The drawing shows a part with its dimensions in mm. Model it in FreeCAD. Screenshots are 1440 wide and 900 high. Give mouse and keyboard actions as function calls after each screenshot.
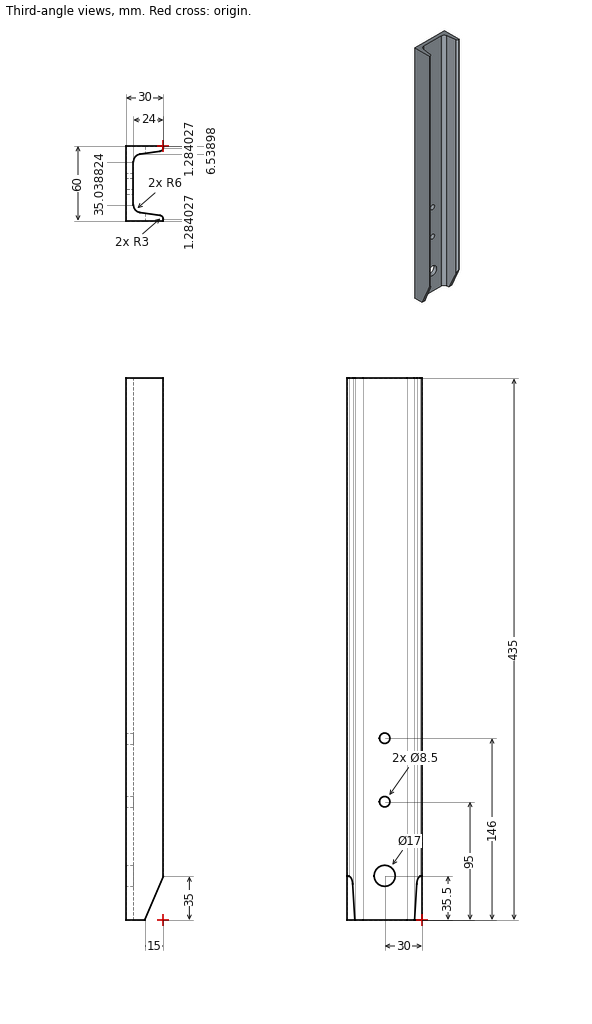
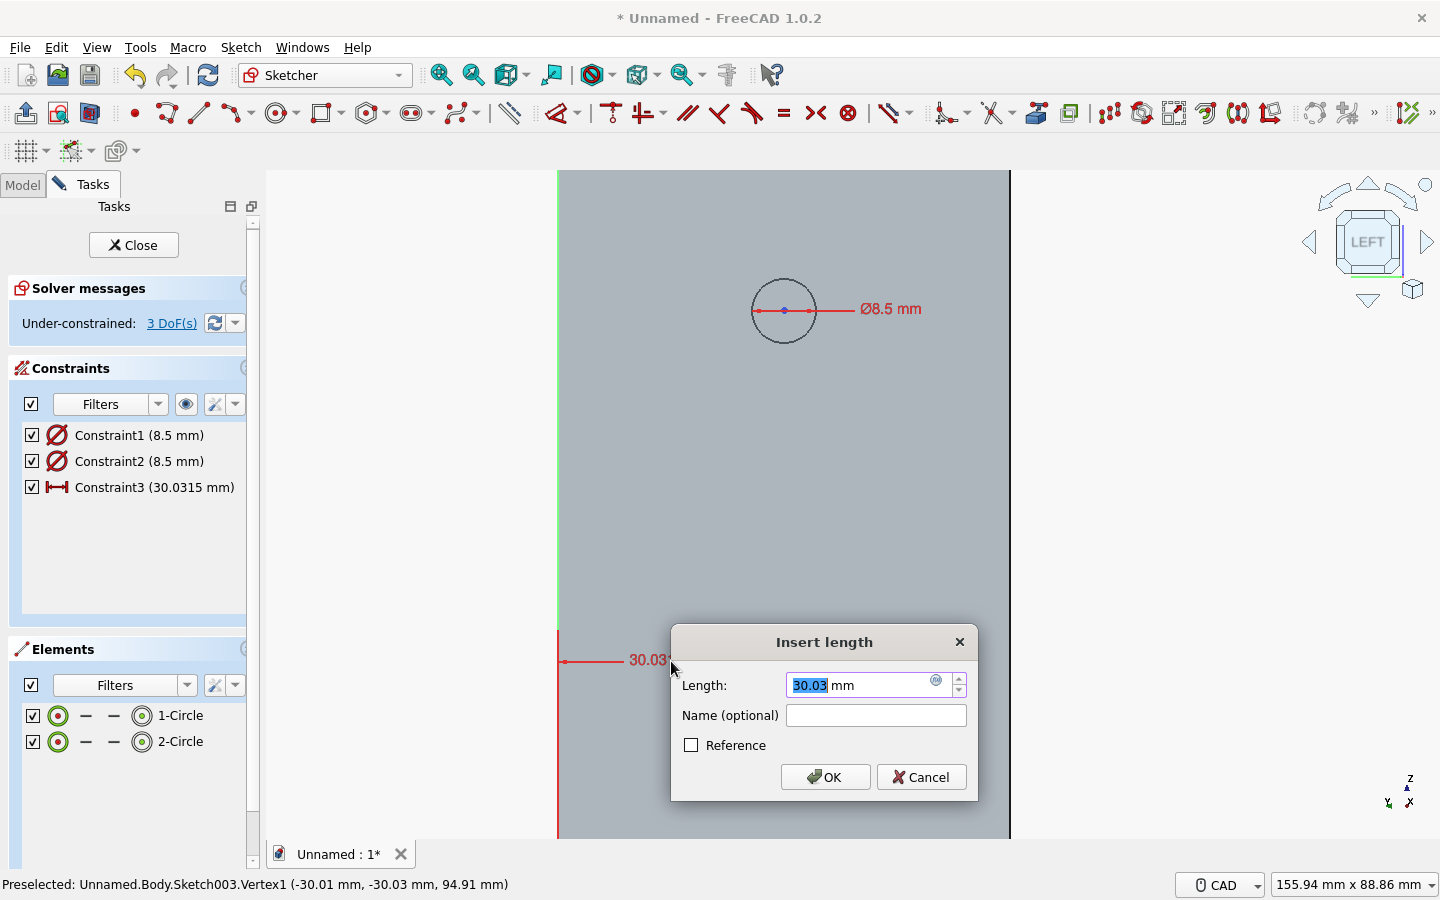
text(30)
key(Return)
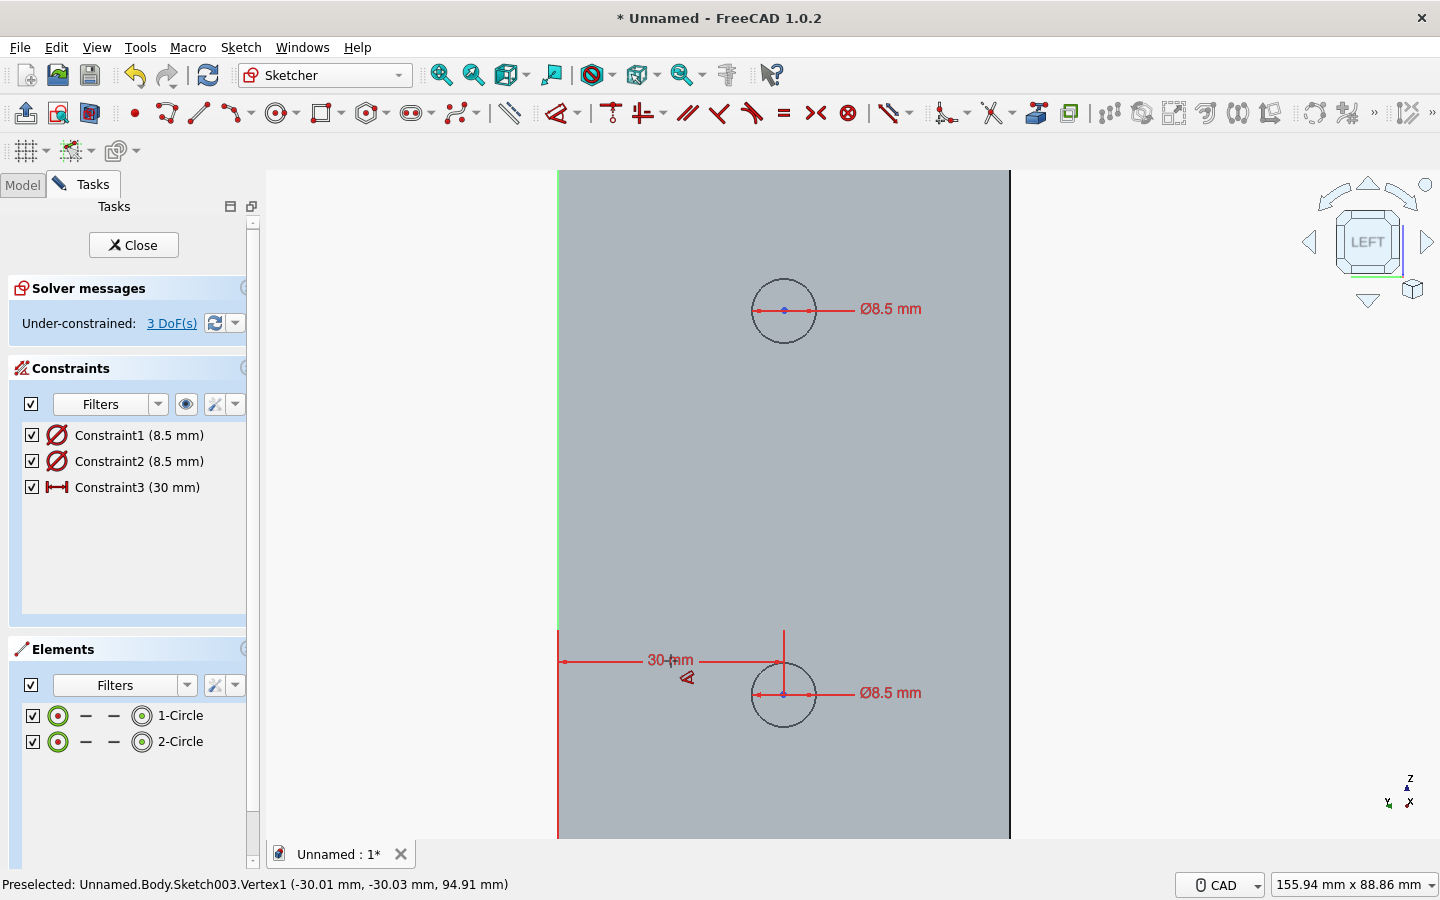
click(784, 695)
click(524, 753)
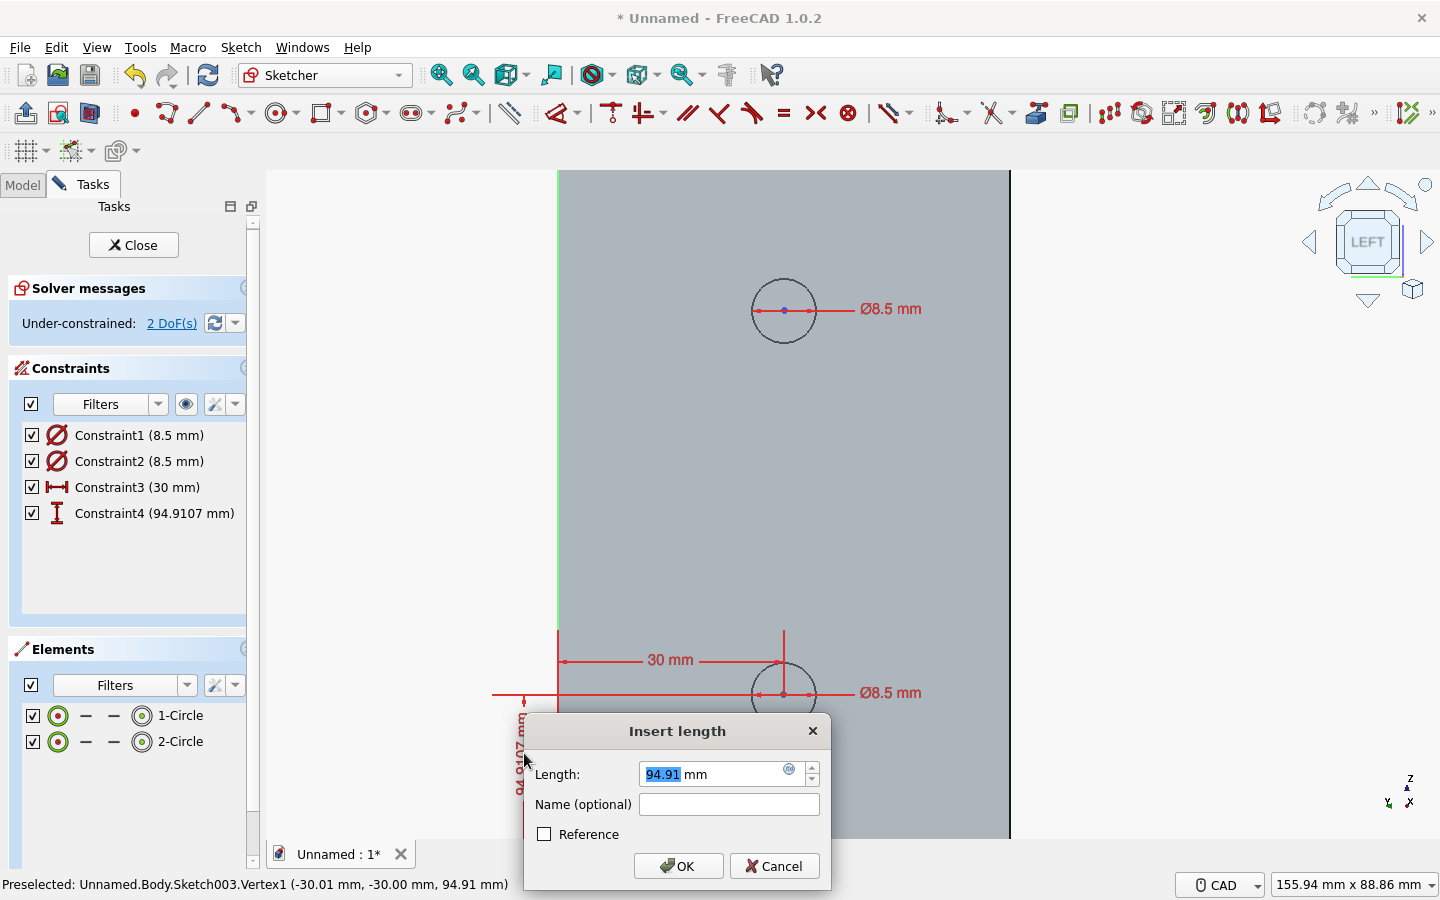
text(95)
key(Return)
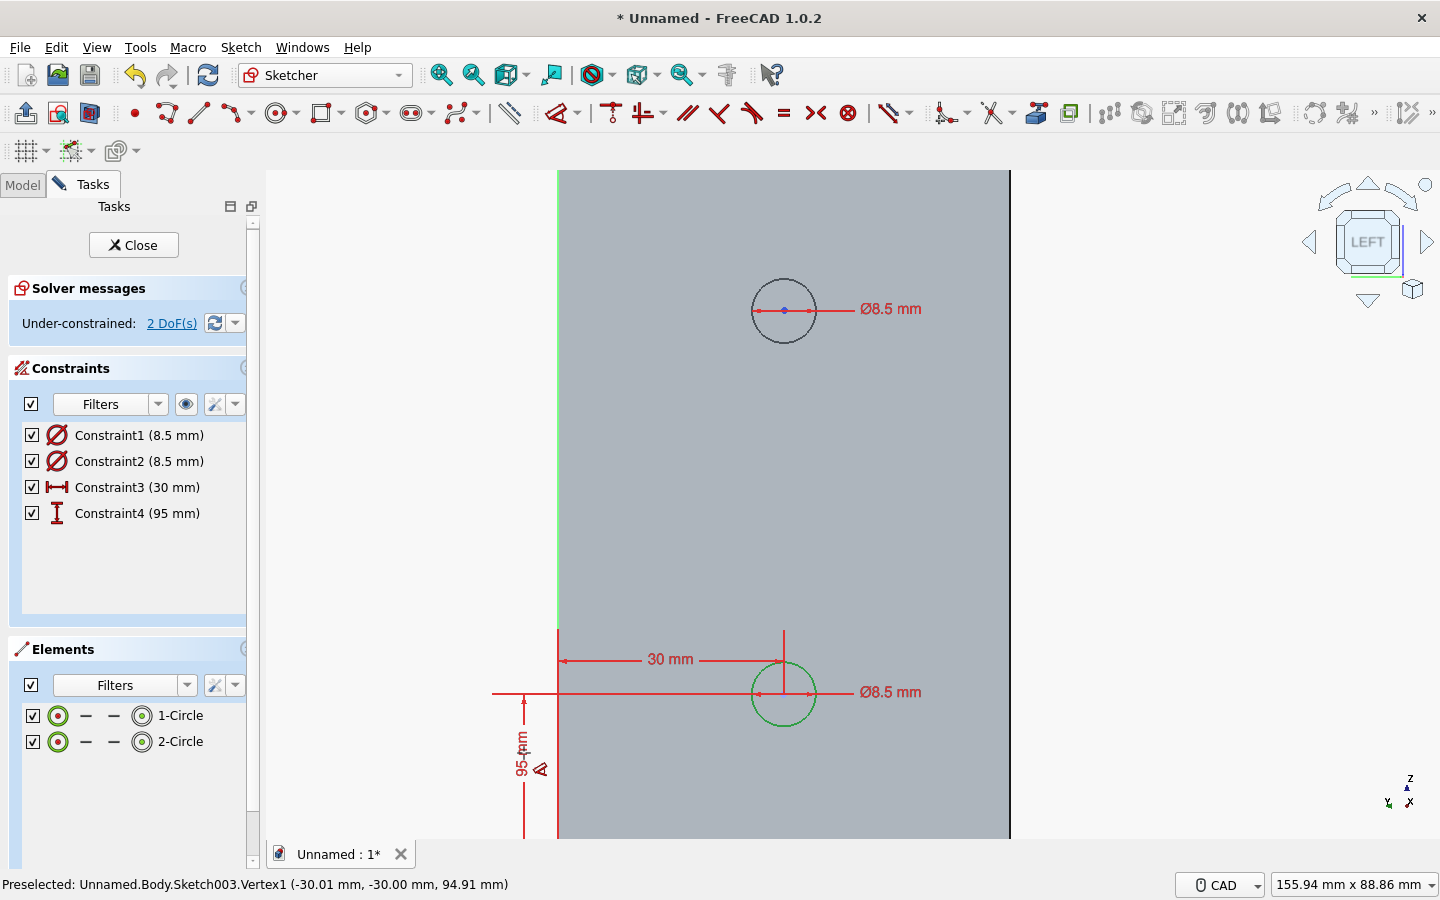
click(784, 311)
click(671, 277)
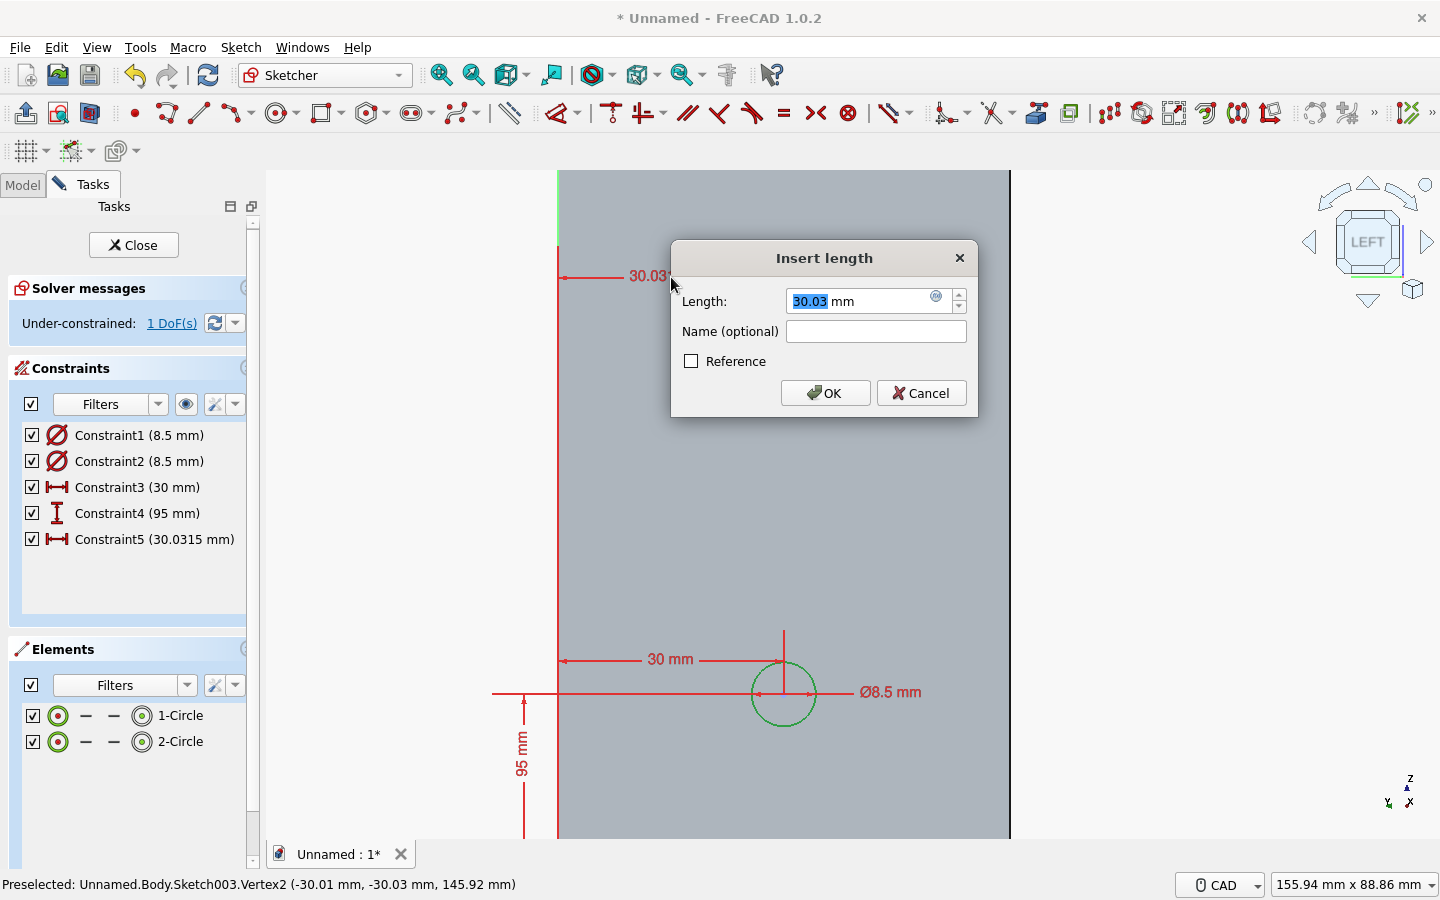
text(30)
key(Return)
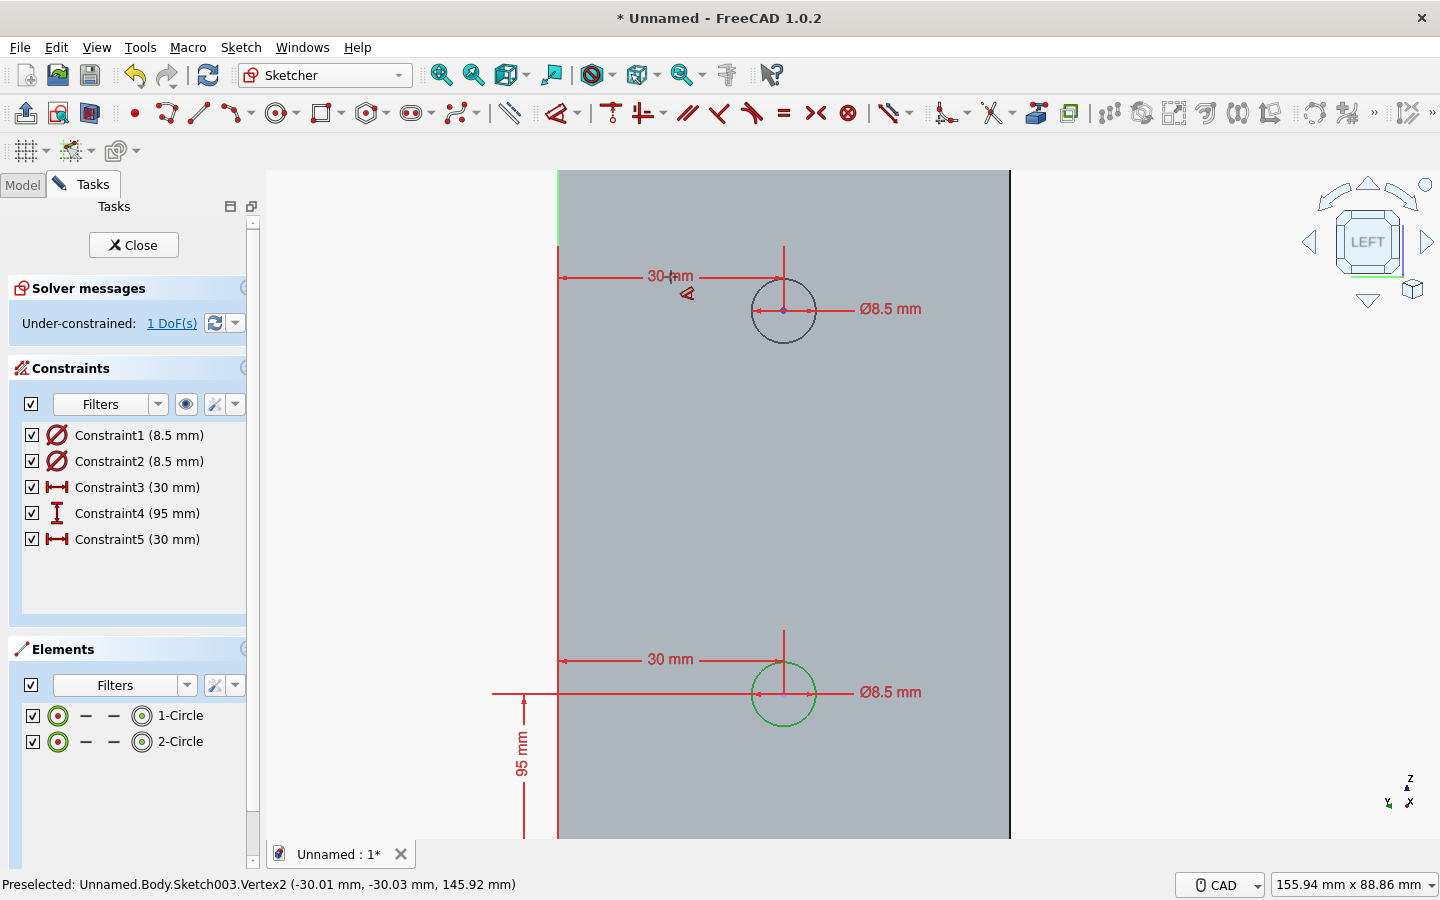
click(784, 311)
click(524, 561)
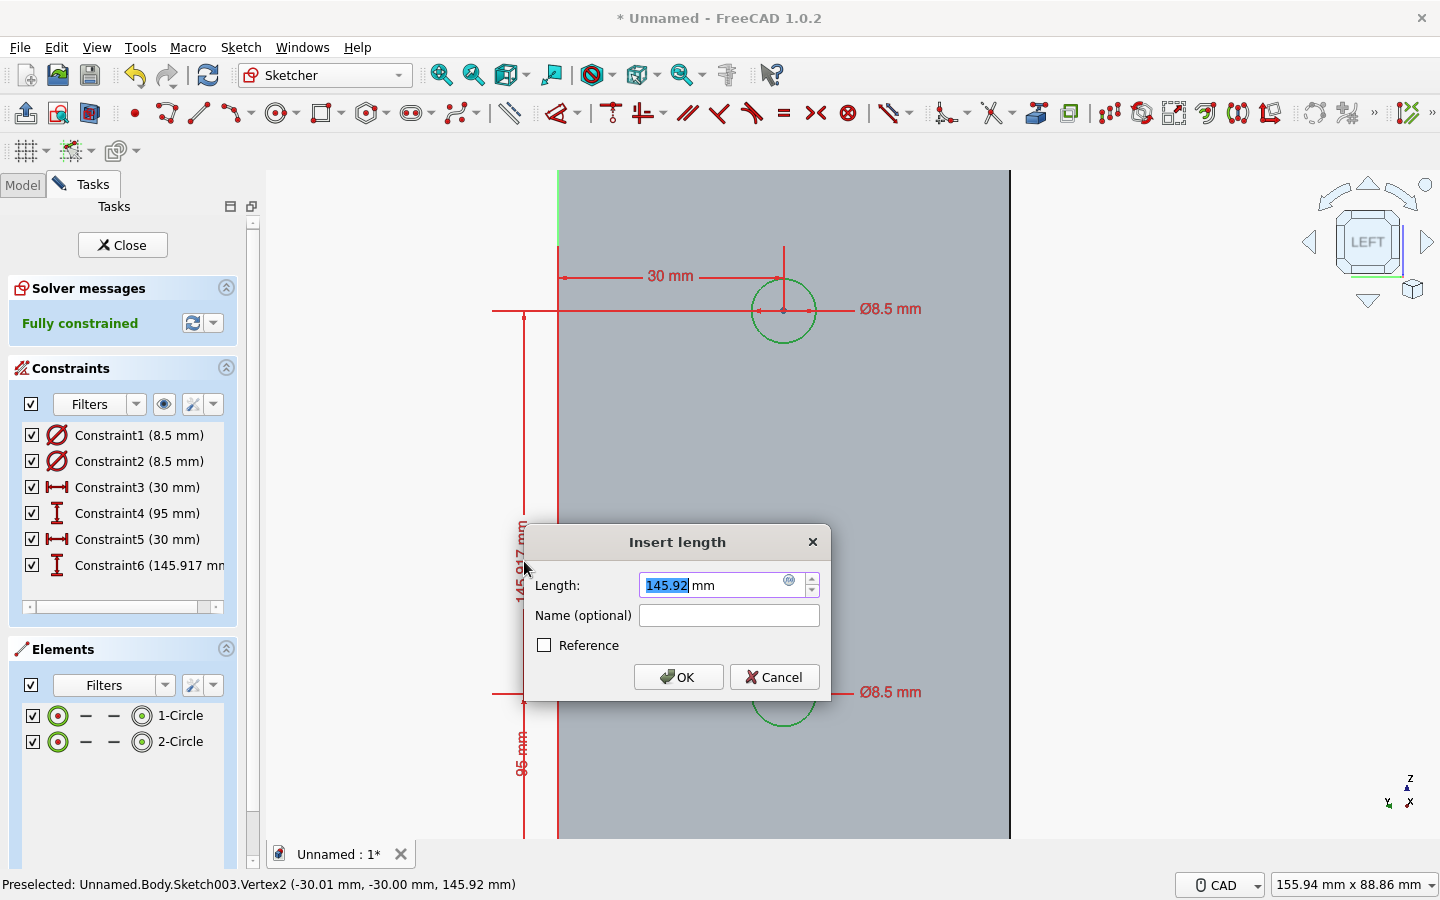
text(146)
key(Return)
key(Escape)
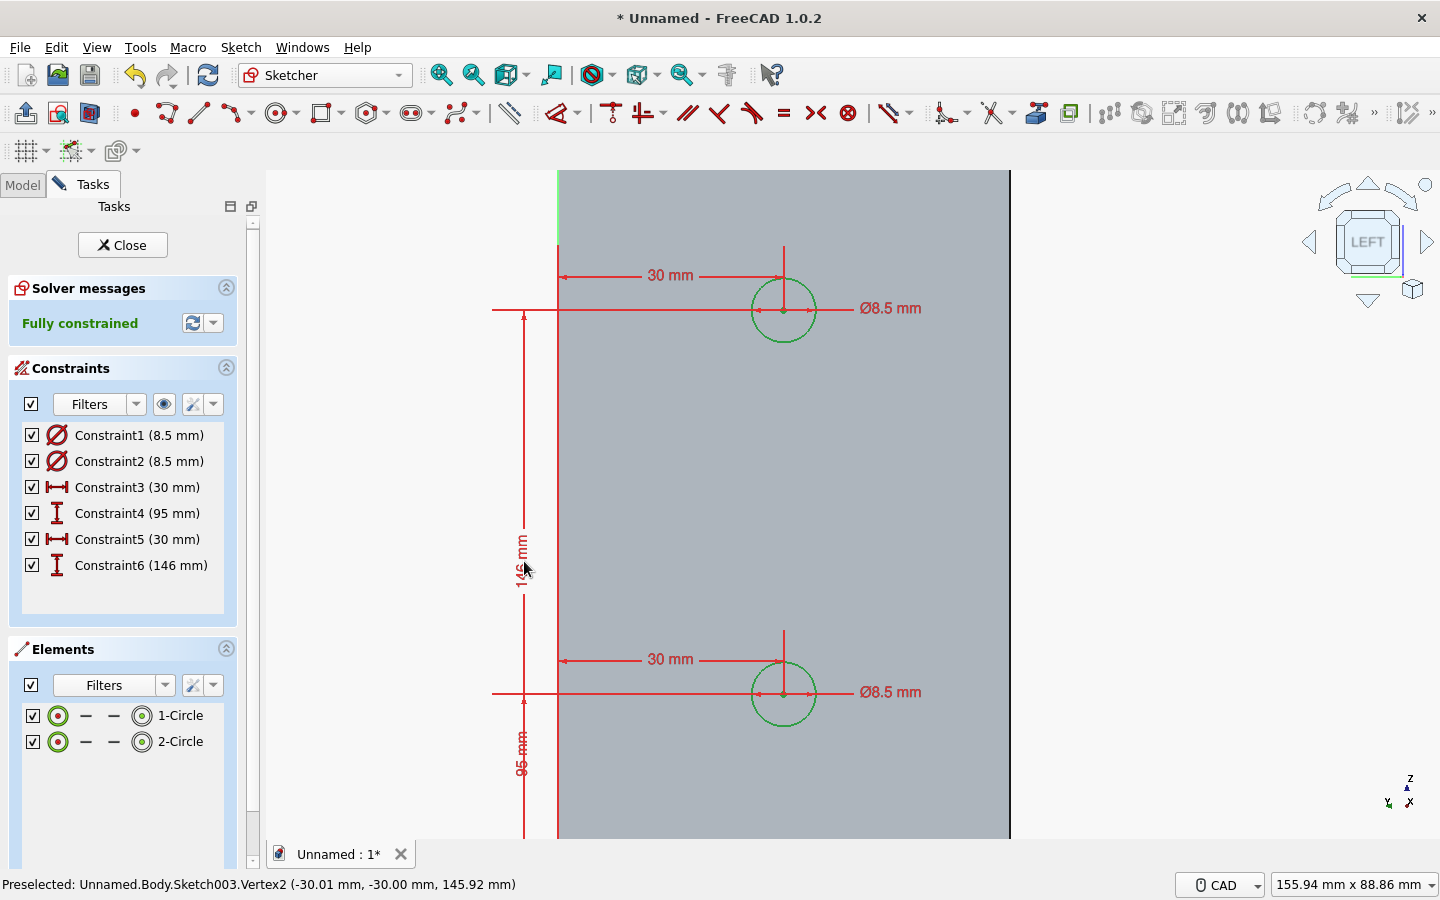
click(123, 245)